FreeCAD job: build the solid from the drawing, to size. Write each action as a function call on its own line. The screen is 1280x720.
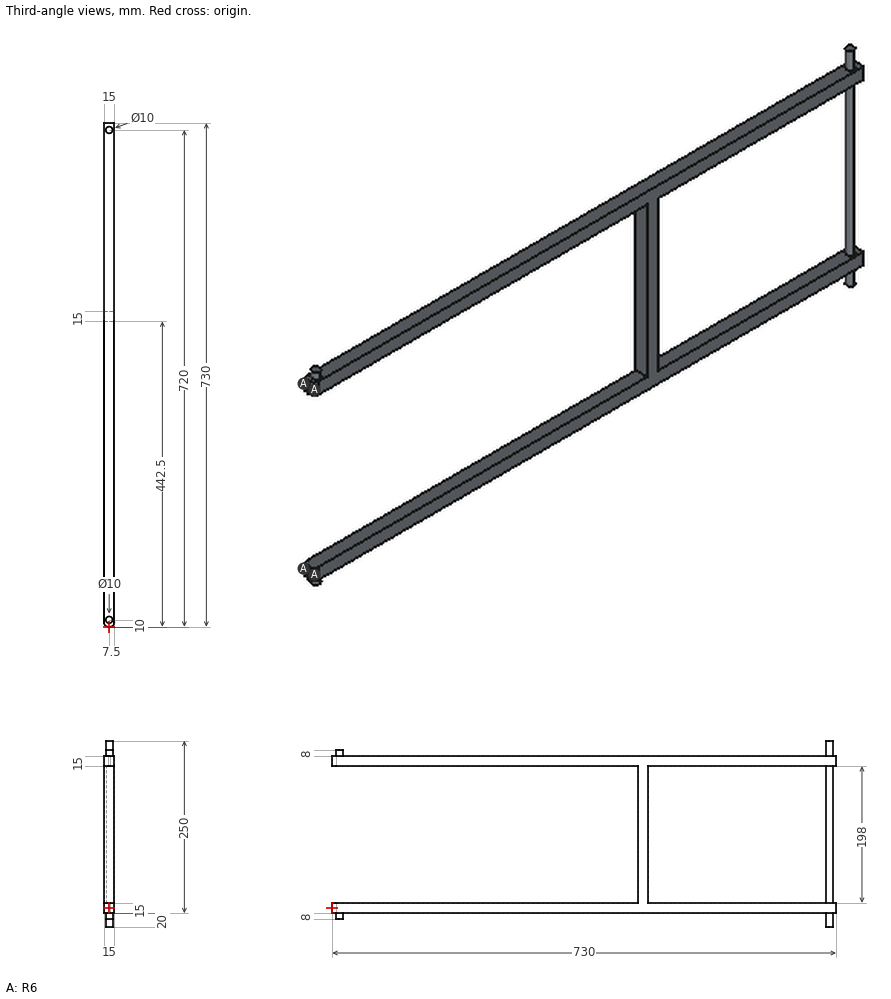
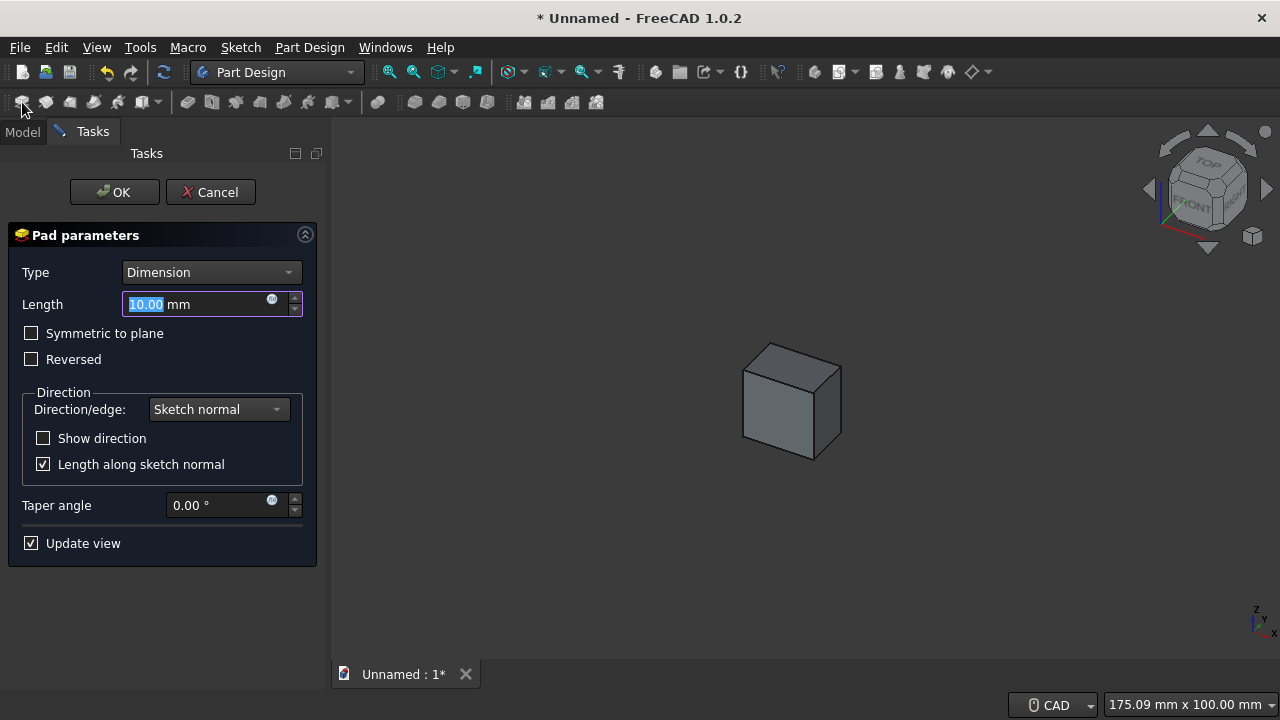
text(730)
key(Tab)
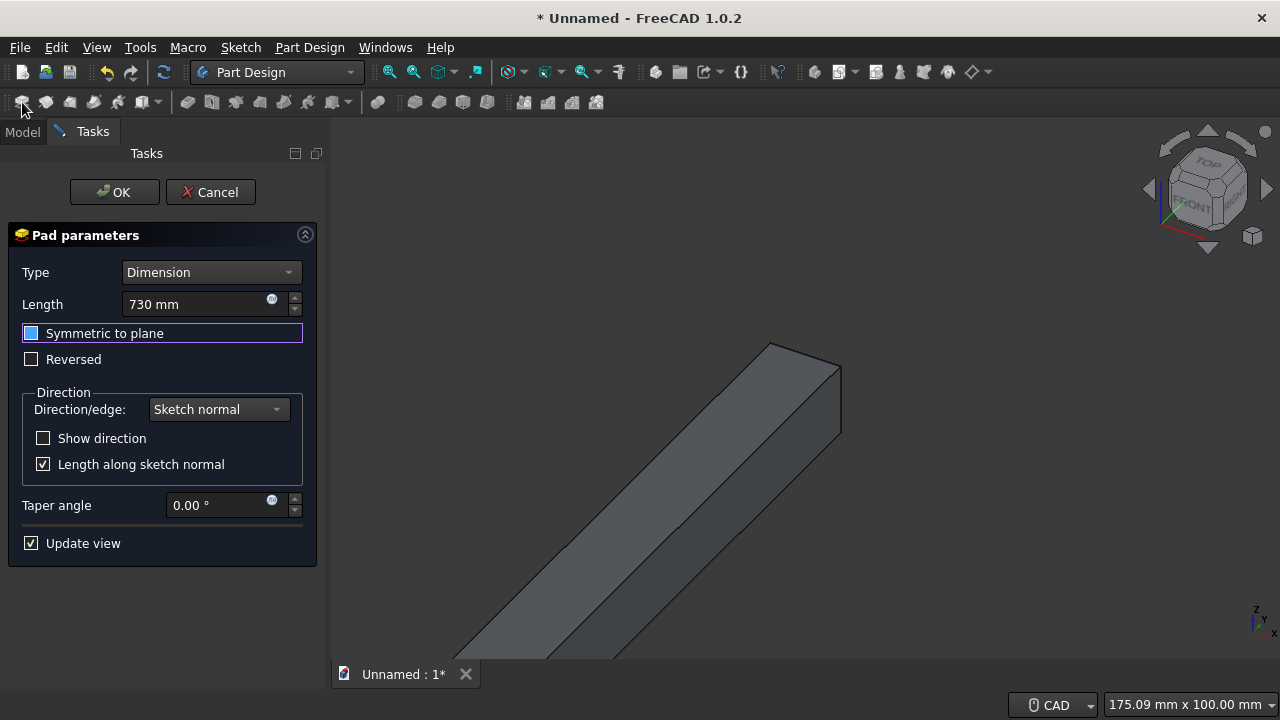
click(30, 359)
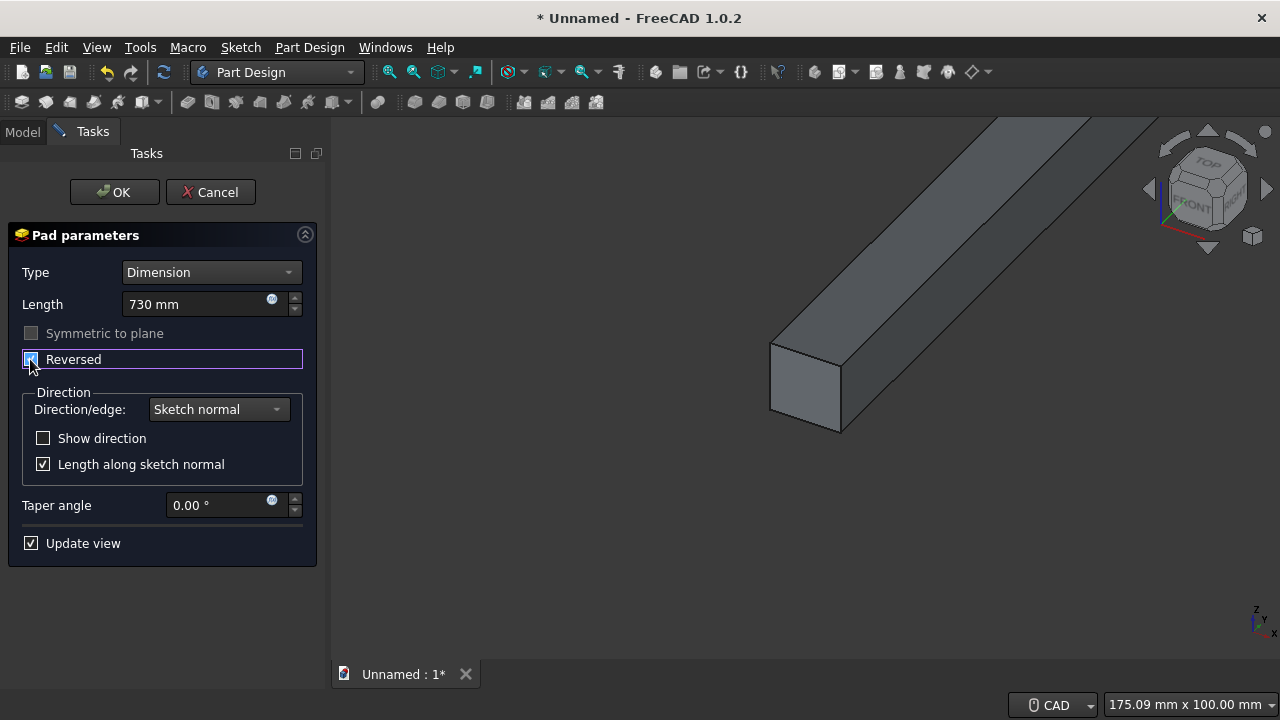
click(115, 192)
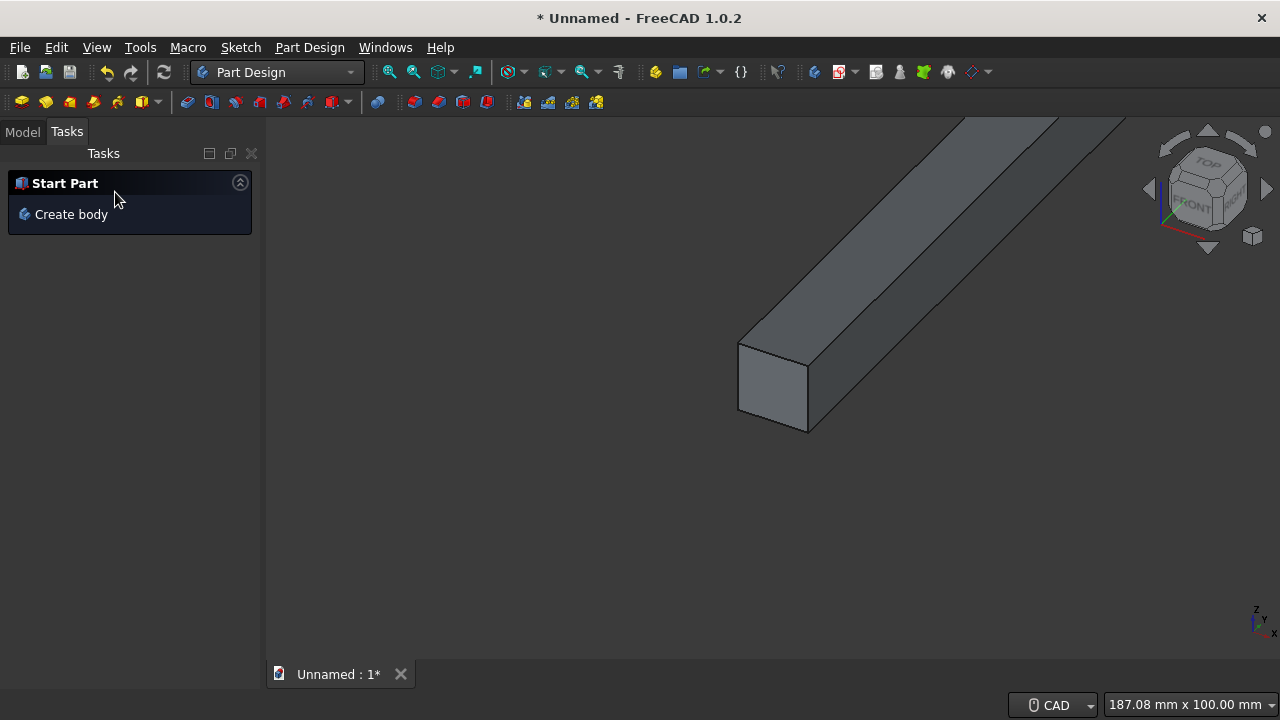
click(390, 72)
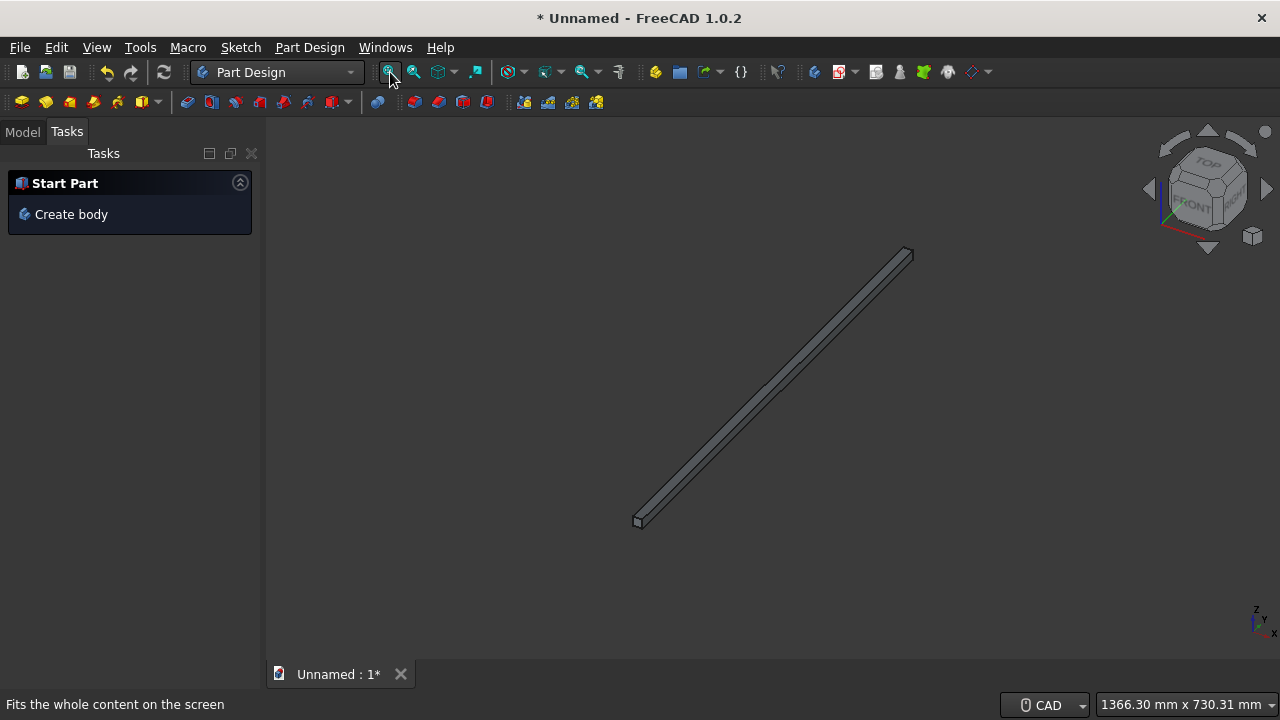
key(5)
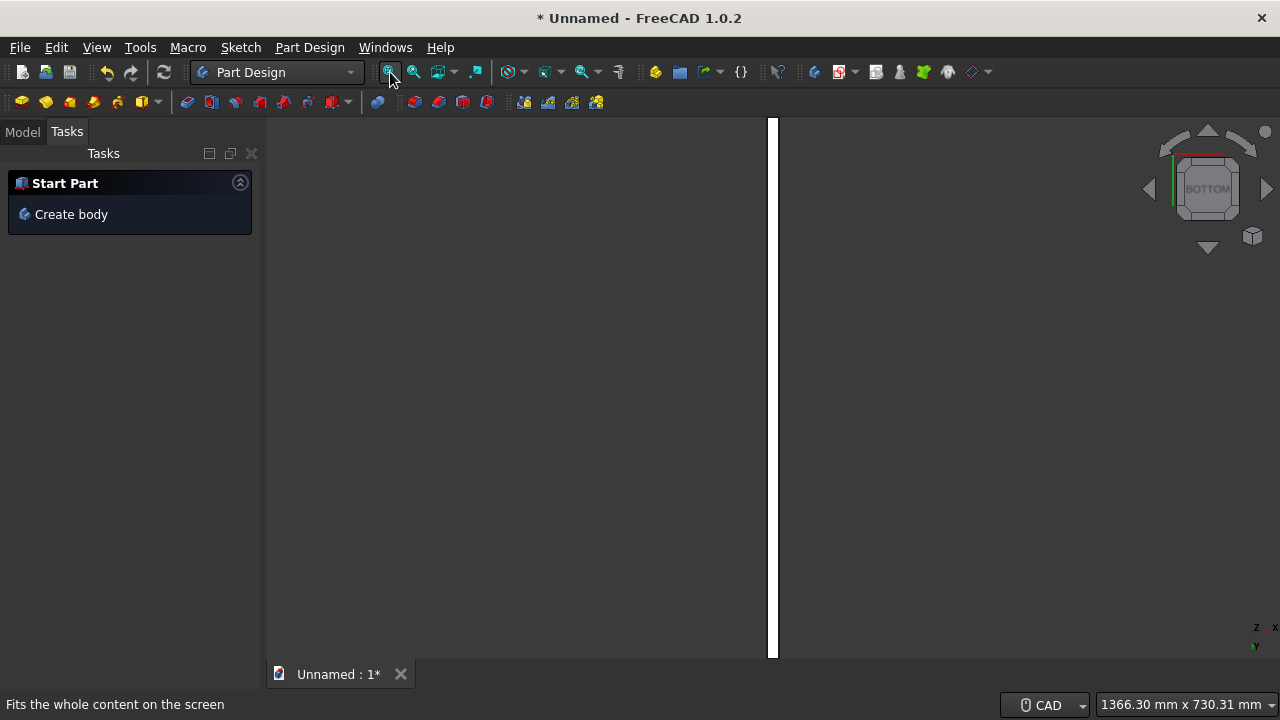
click(390, 72)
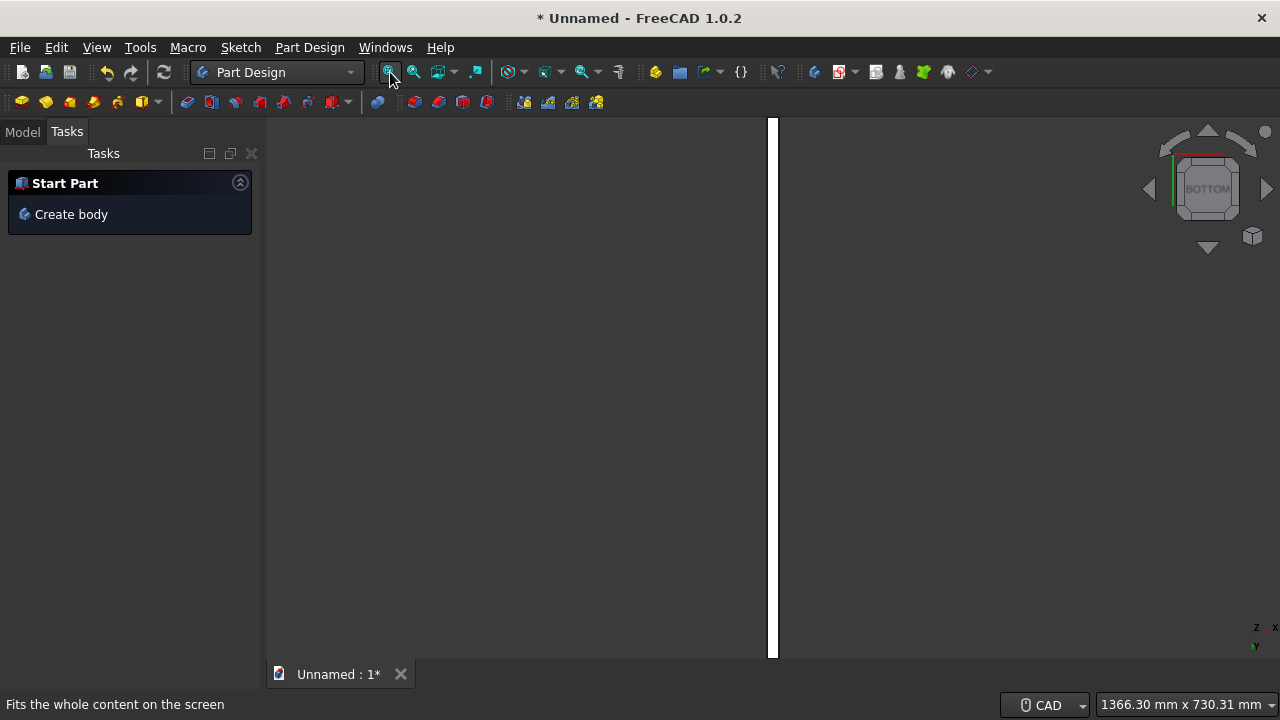
scroll(773, 619, up, 4)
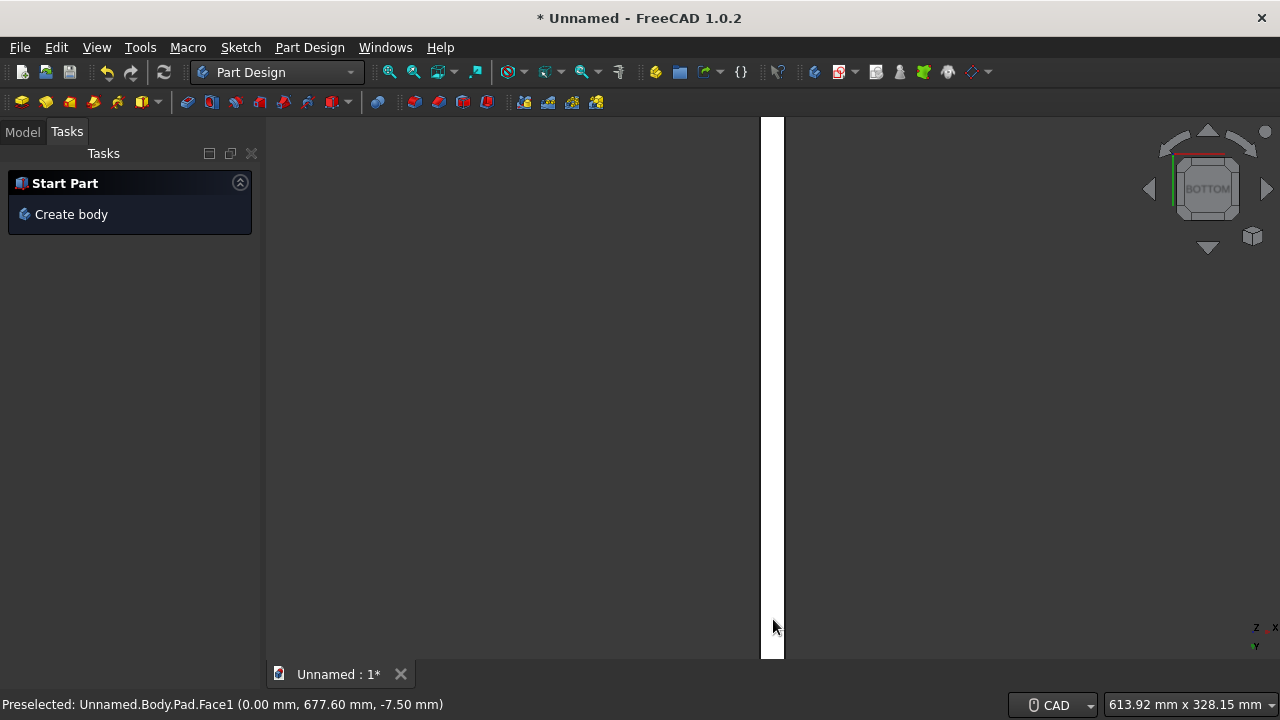
click(772, 620)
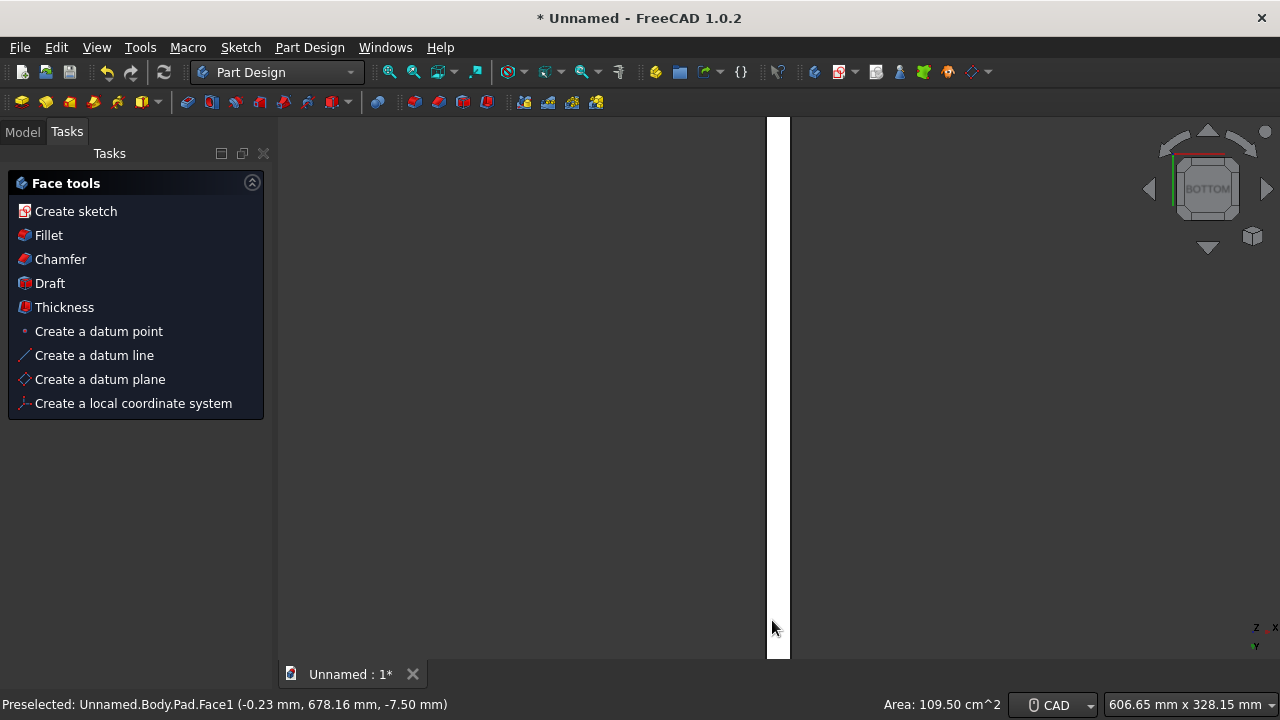
click(840, 72)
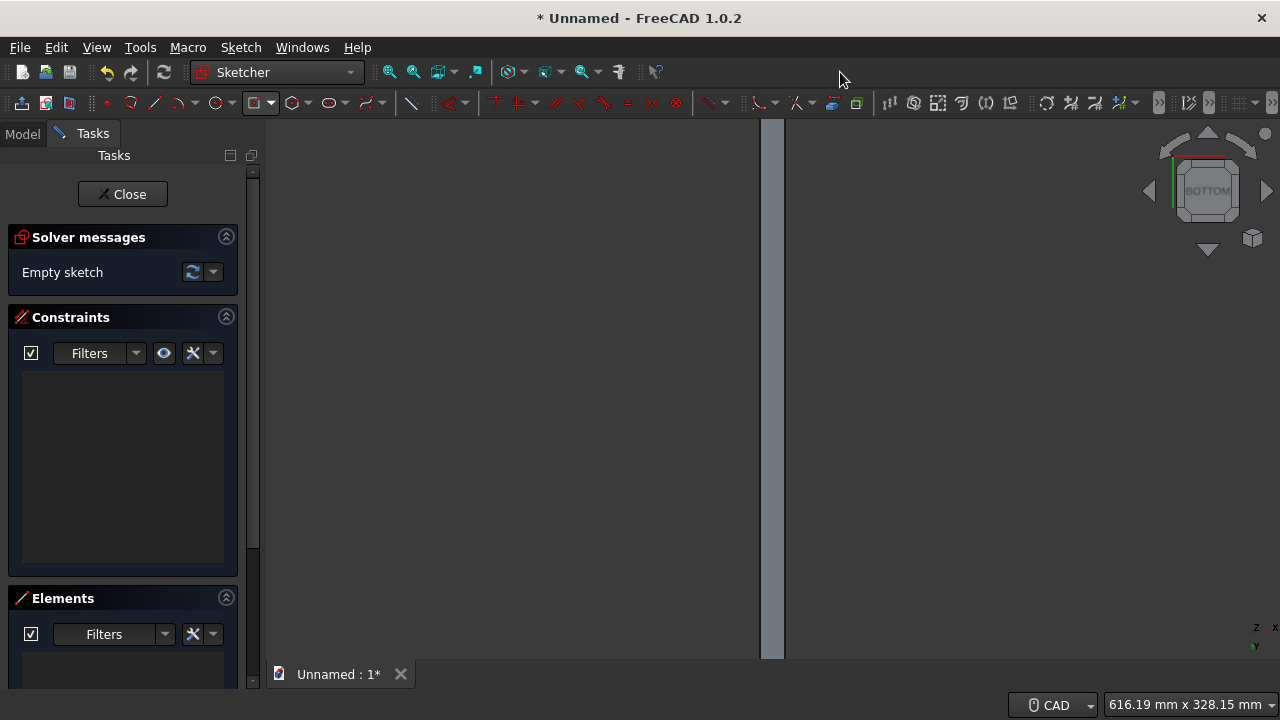
scroll(704, 389, down, 5)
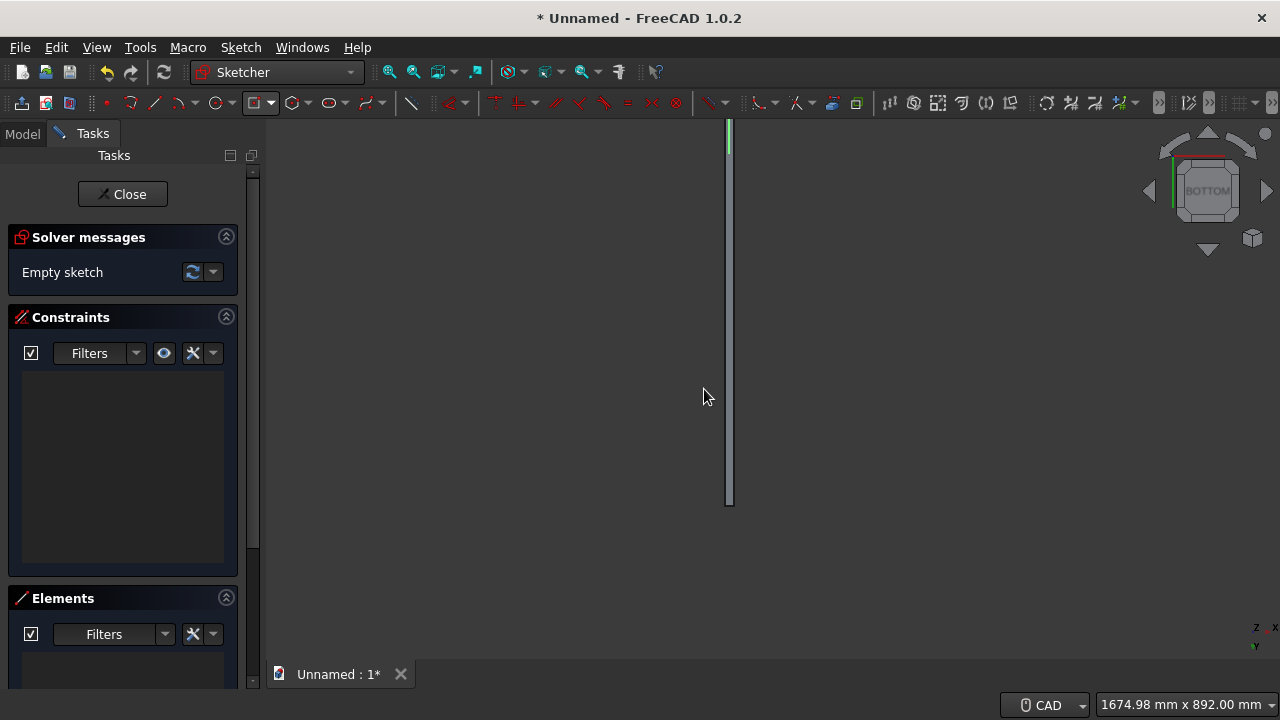
scroll(704, 389, down, 5)